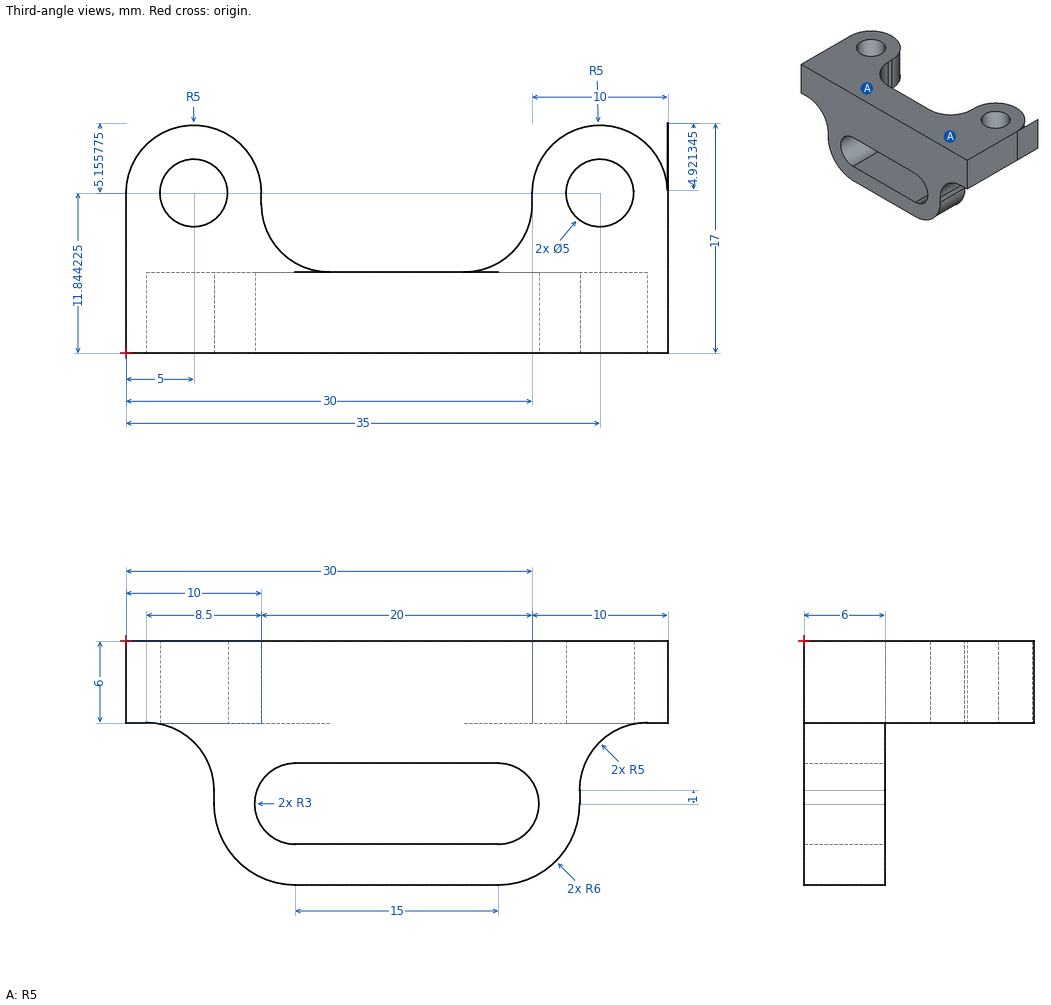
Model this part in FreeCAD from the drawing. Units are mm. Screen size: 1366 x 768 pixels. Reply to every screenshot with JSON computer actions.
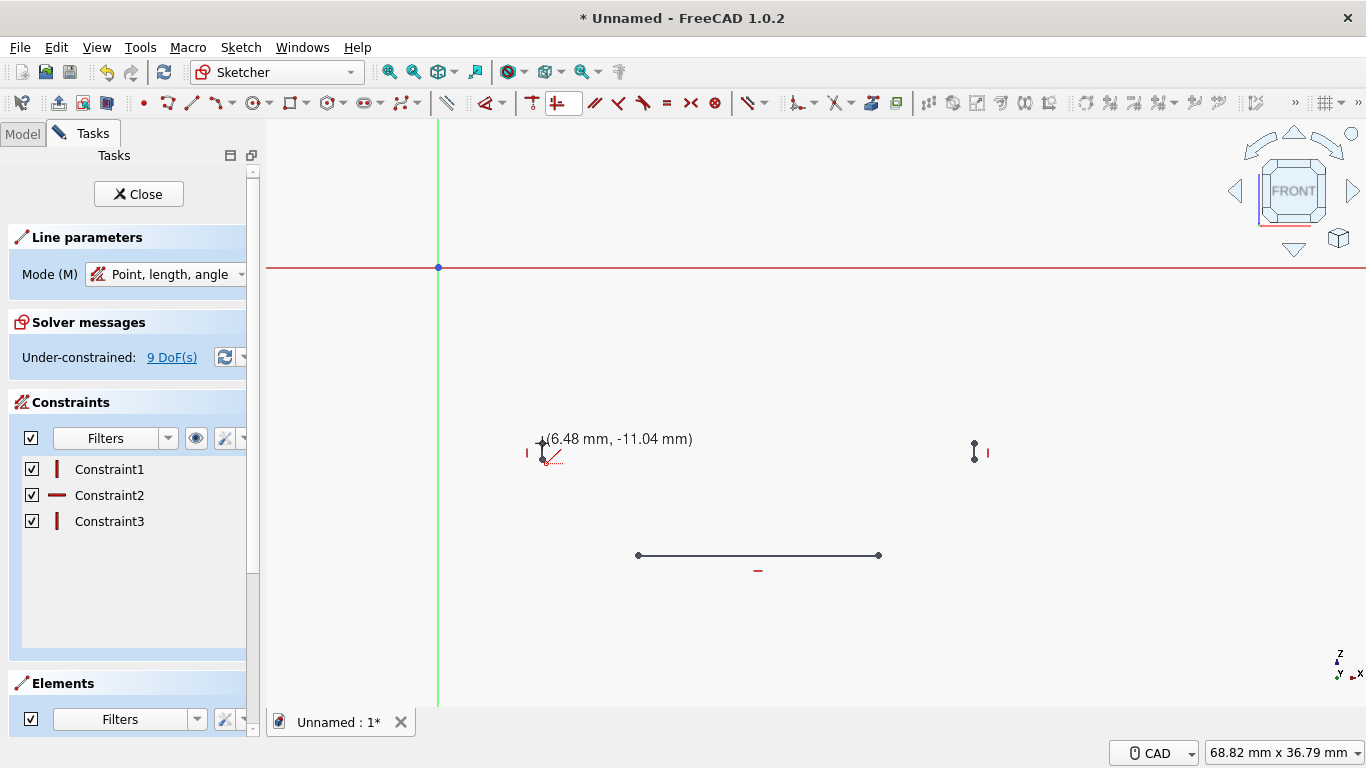
{"action": "key", "text": "g m"}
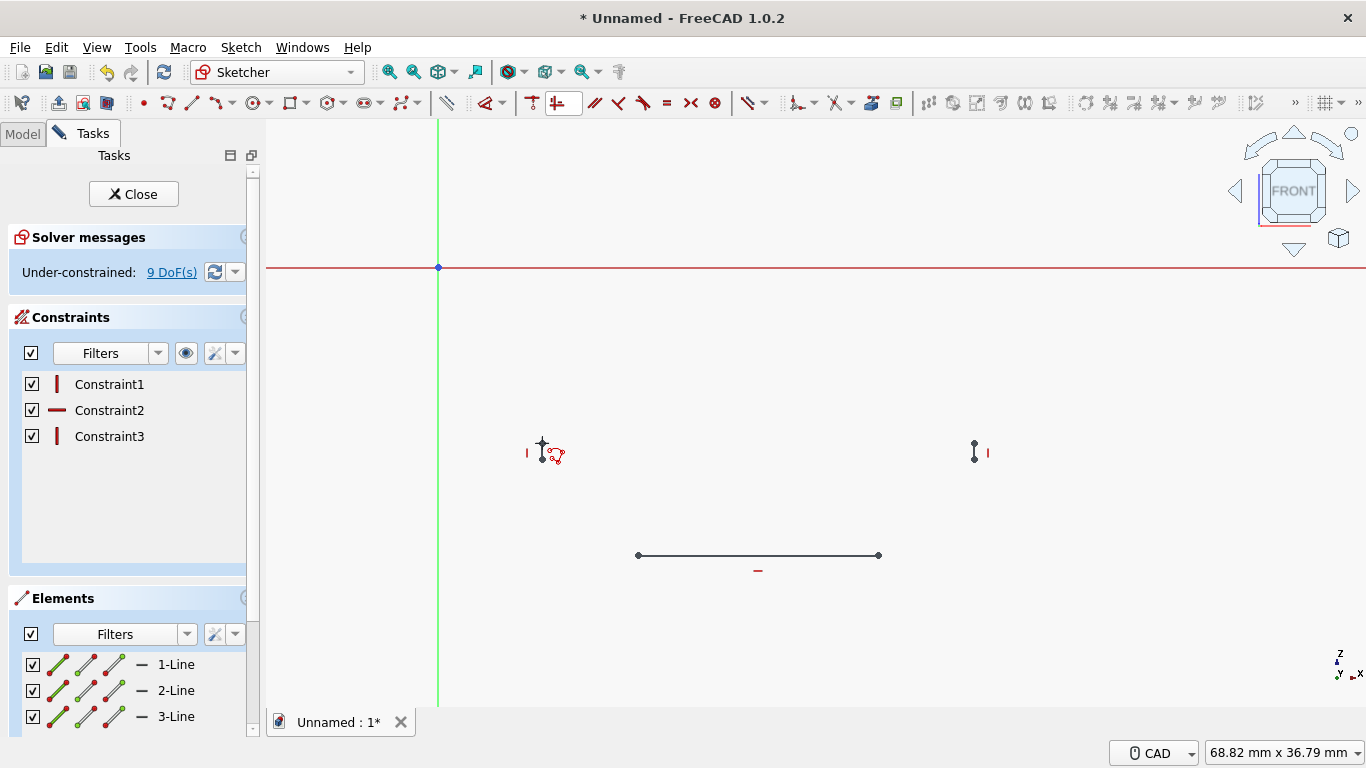
{"action": "left_click", "coordinate": [462, 363]}
{"action": "left_click", "coordinate": [598, 363]}
{"action": "left_click", "coordinate": [598, 268]}
{"action": "left_click", "coordinate": [918, 277]}
{"action": "left_click", "coordinate": [918, 363]}
{"action": "left_click", "coordinate": [1054, 363]}
{"action": "right_click", "coordinate": [1054, 363]}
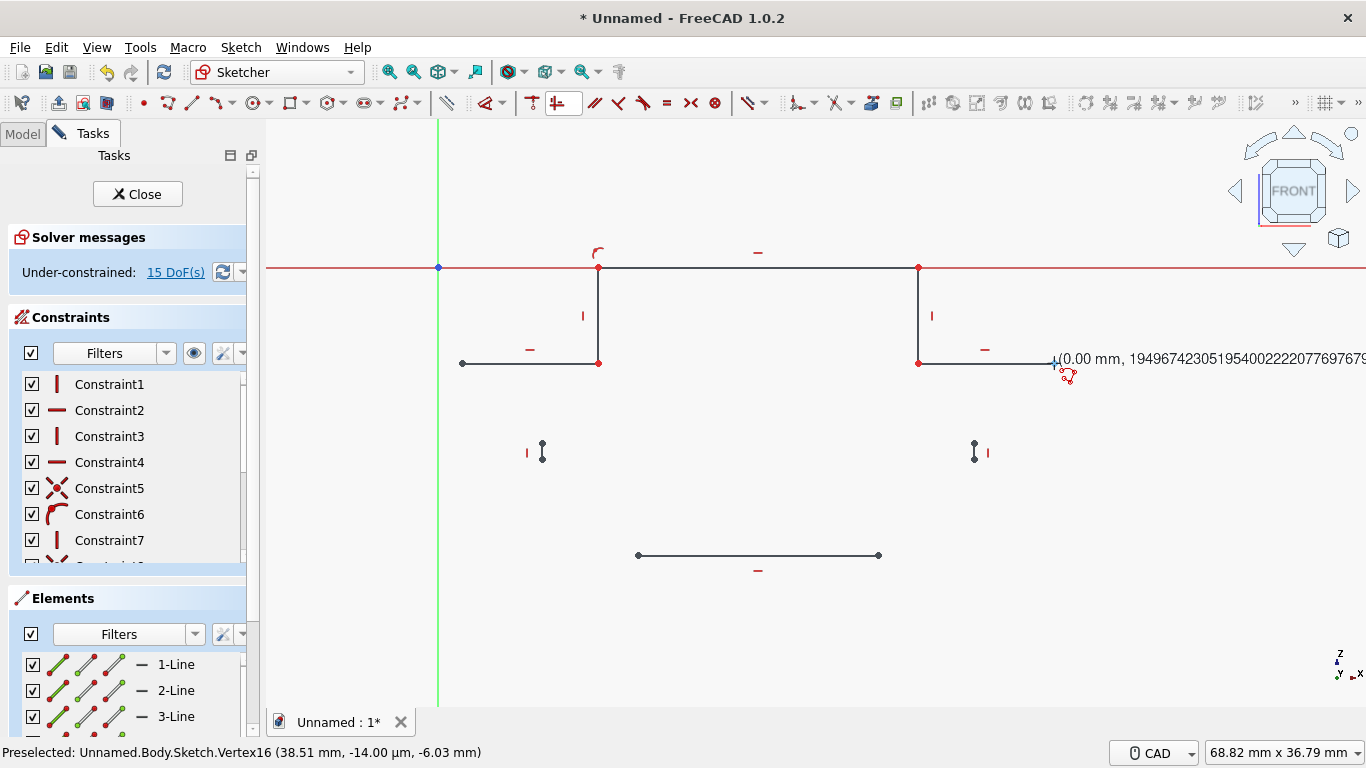
{"action": "key", "text": "g 3 a"}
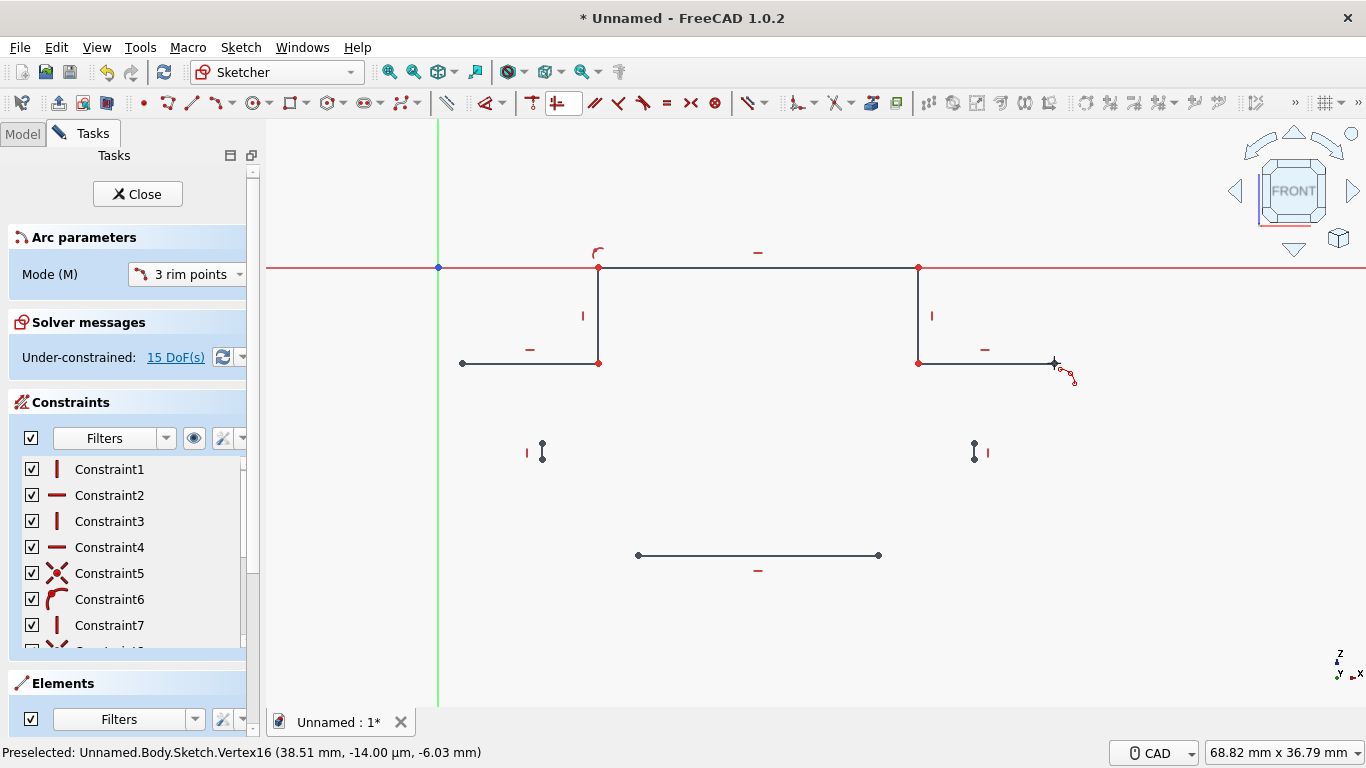
{"action": "scroll", "coordinate": [974, 459], "scroll_direction": "up", "scroll_amount": 4}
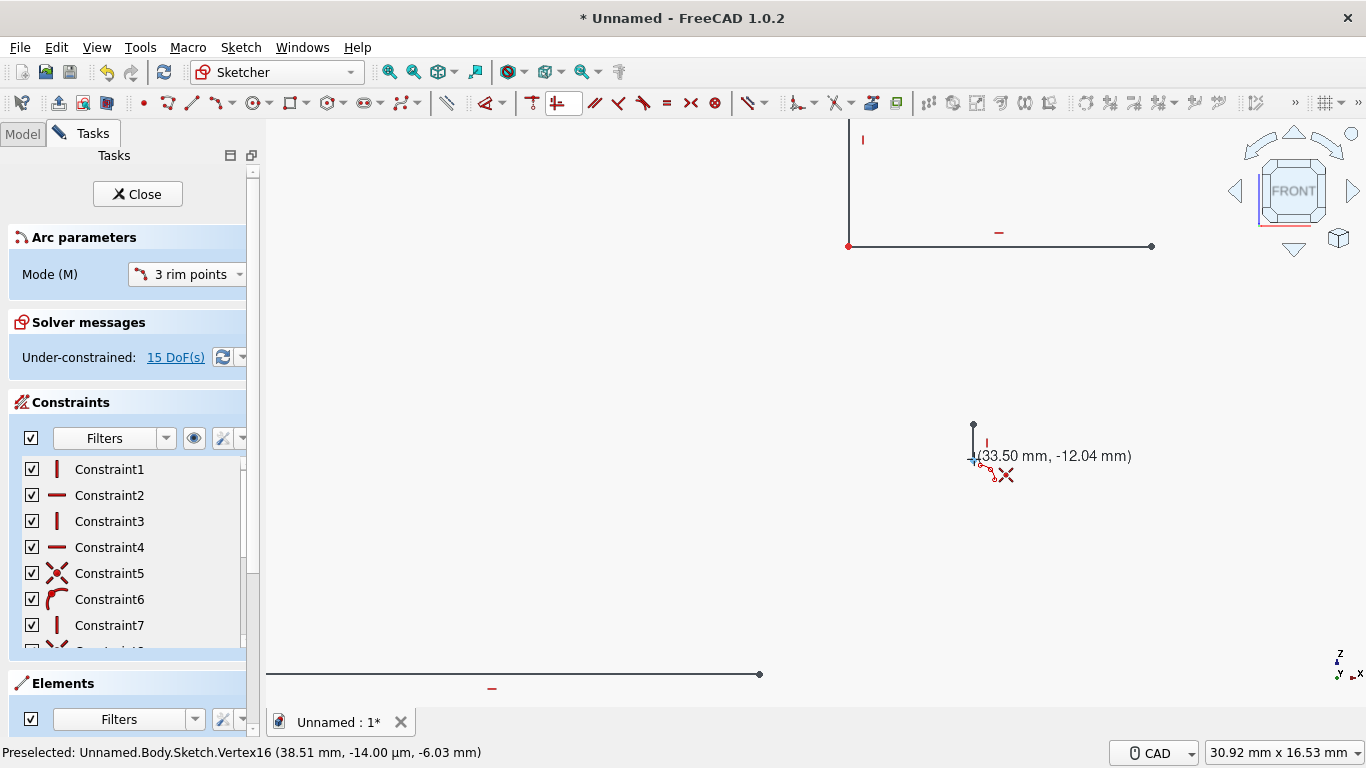
{"action": "left_click", "coordinate": [973, 461]}
{"action": "left_click", "coordinate": [760, 674]}
{"action": "left_click", "coordinate": [911, 610]}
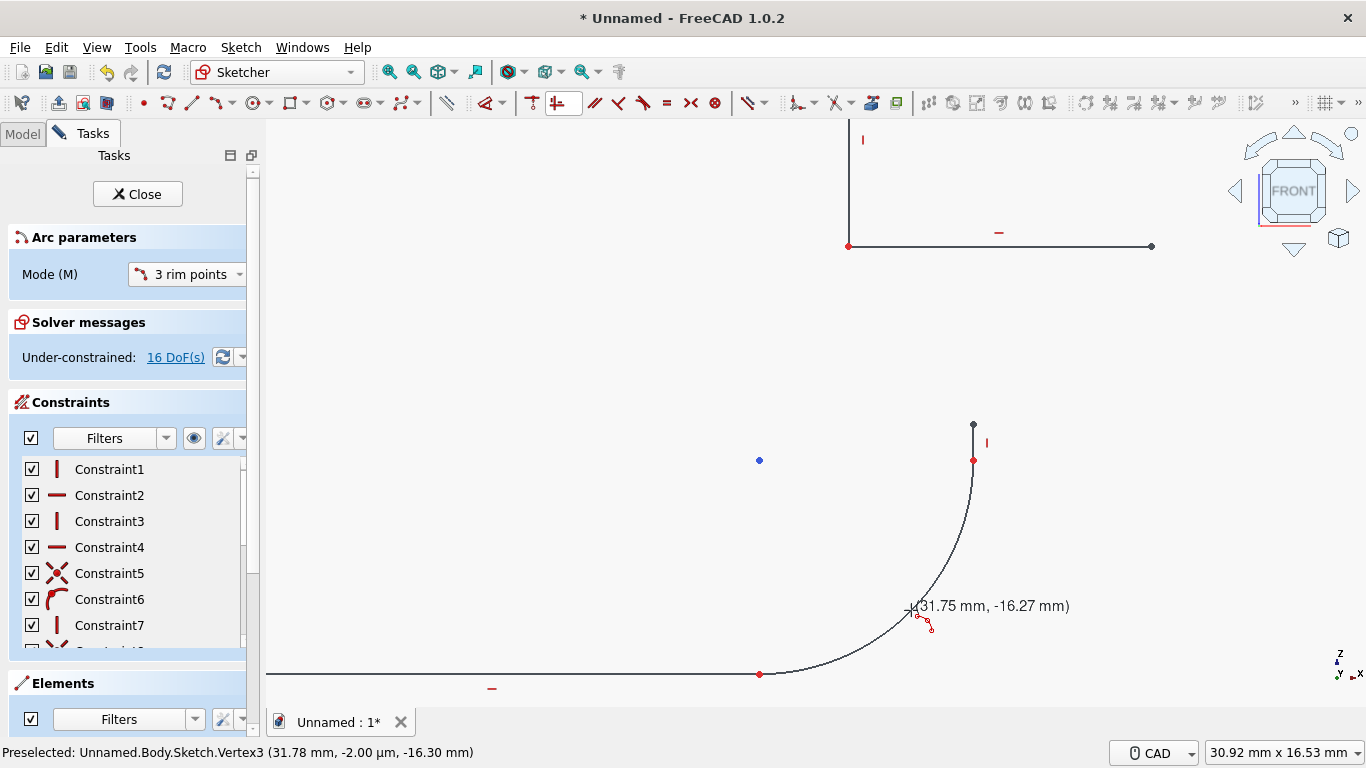
{"action": "scroll", "coordinate": [977, 462], "scroll_direction": "down", "scroll_amount": 4}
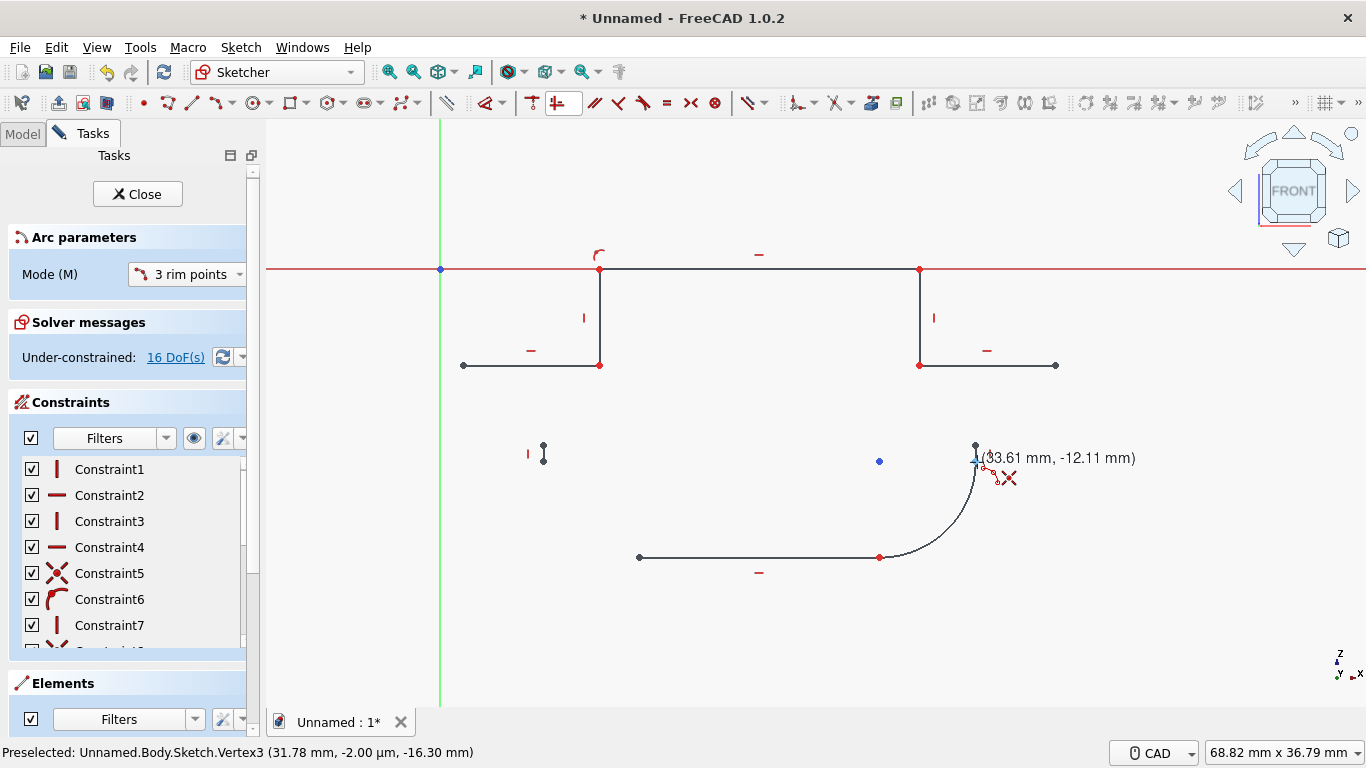
{"action": "left_click", "coordinate": [640, 558]}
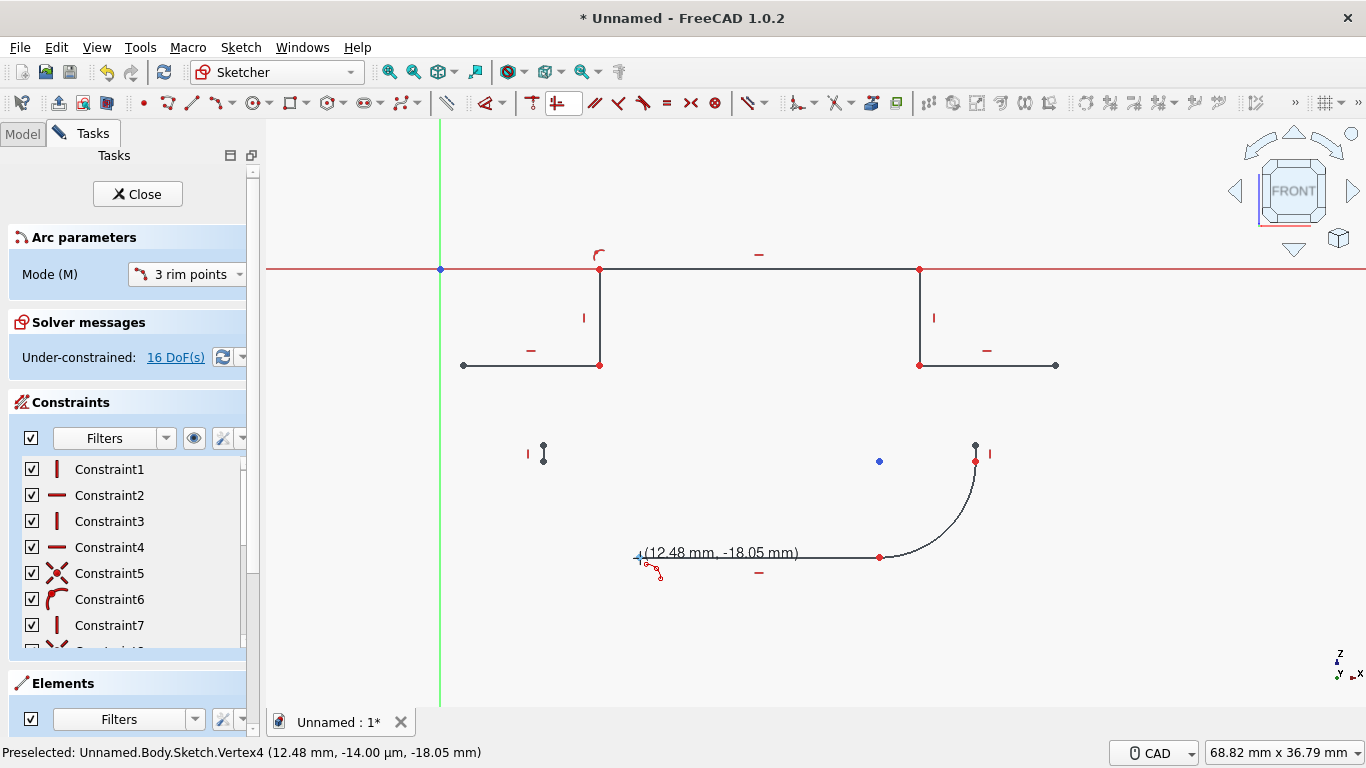
{"action": "scroll", "coordinate": [544, 461], "scroll_direction": "up", "scroll_amount": 4}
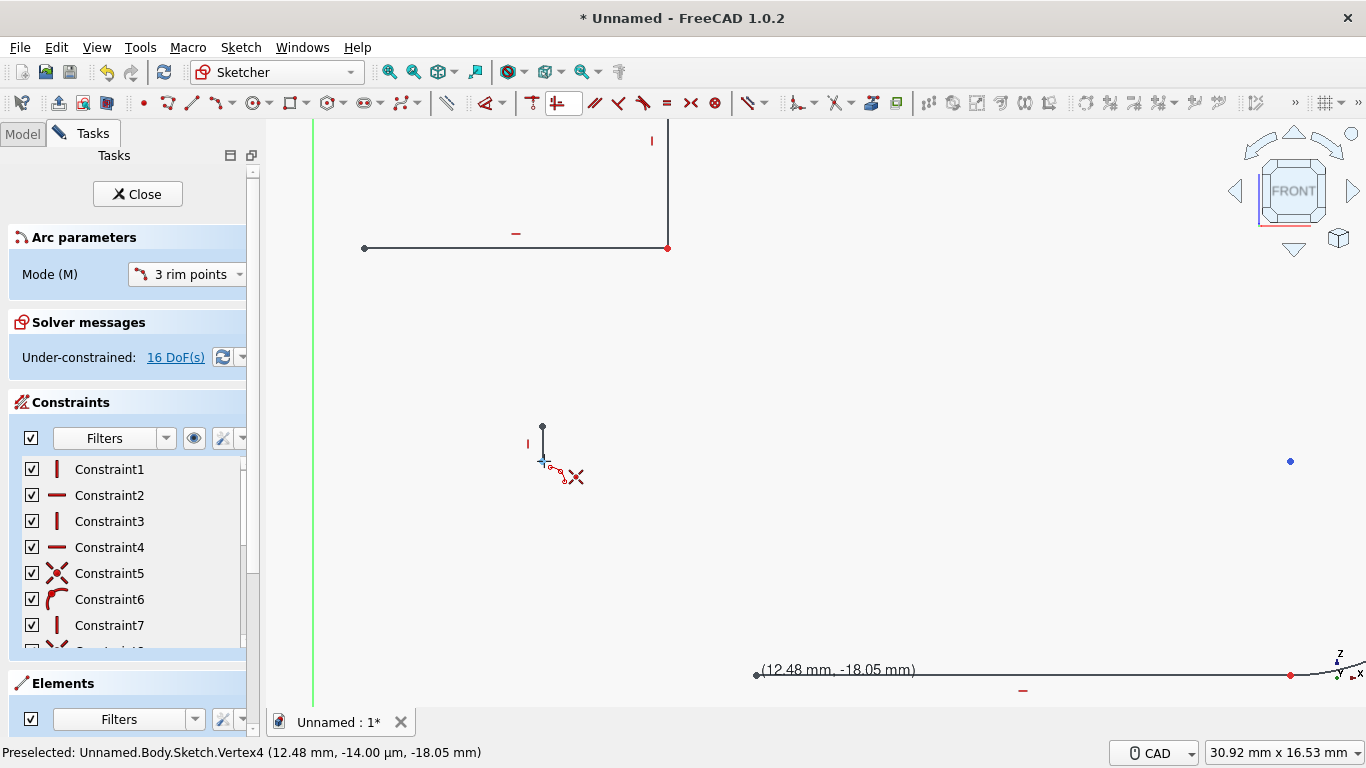
{"action": "left_click", "coordinate": [543, 462]}
{"action": "left_click", "coordinate": [606, 611]}